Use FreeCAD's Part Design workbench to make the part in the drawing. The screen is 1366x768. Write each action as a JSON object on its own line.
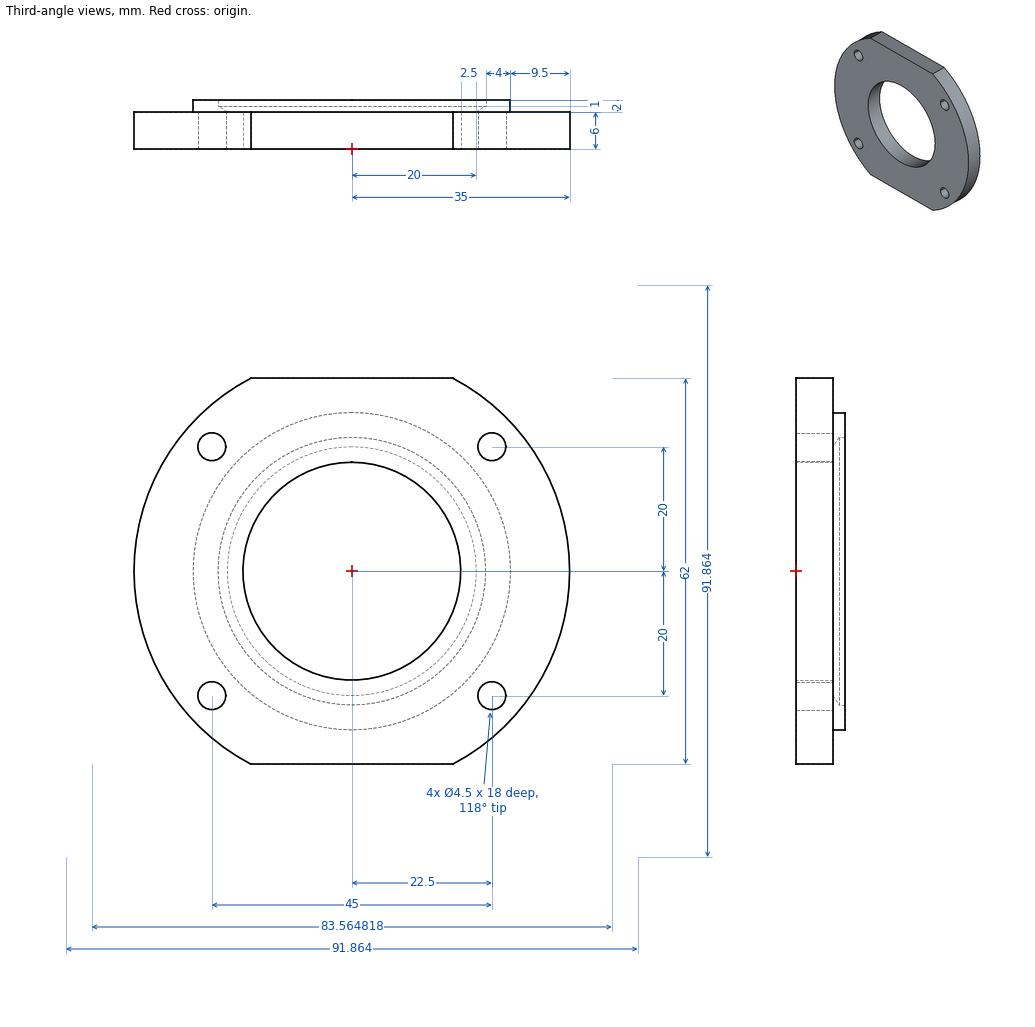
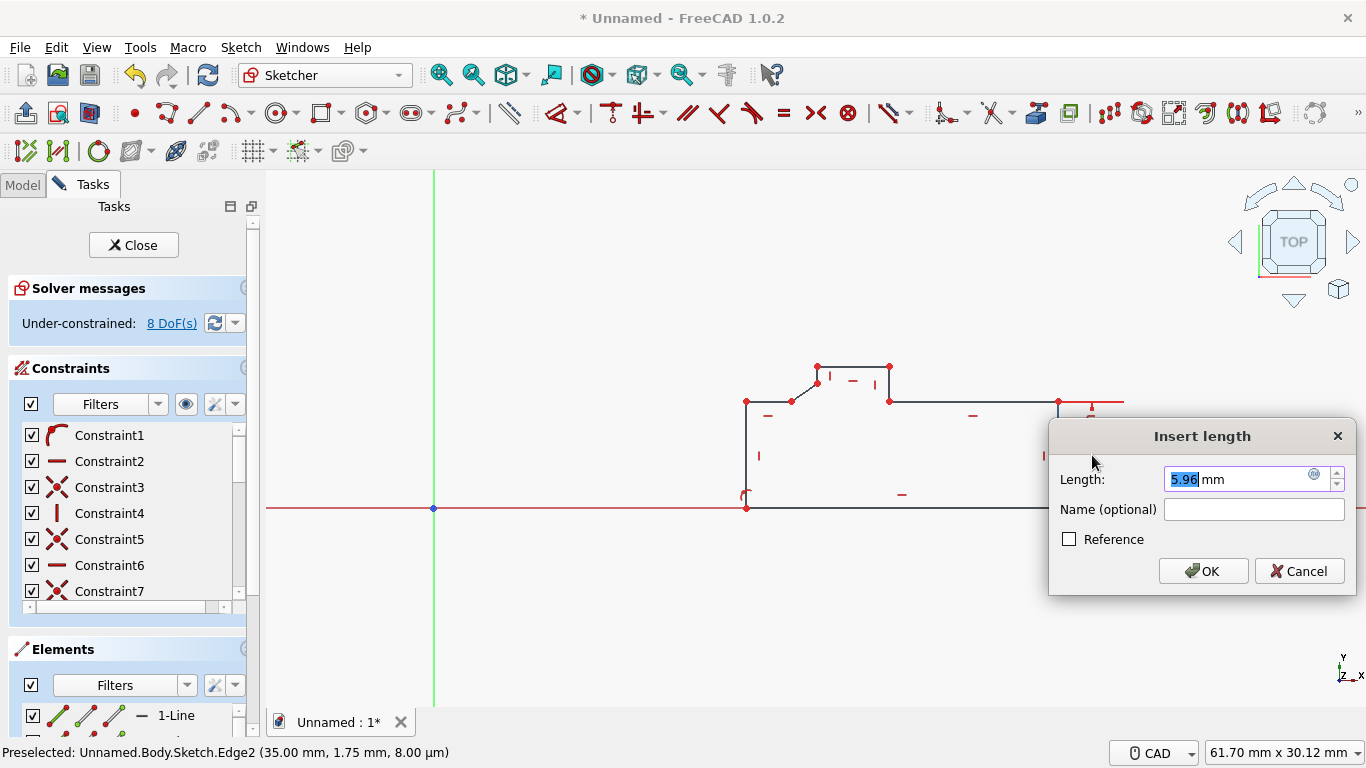
{"action": "type", "text": "6"}
{"action": "key", "text": "Return"}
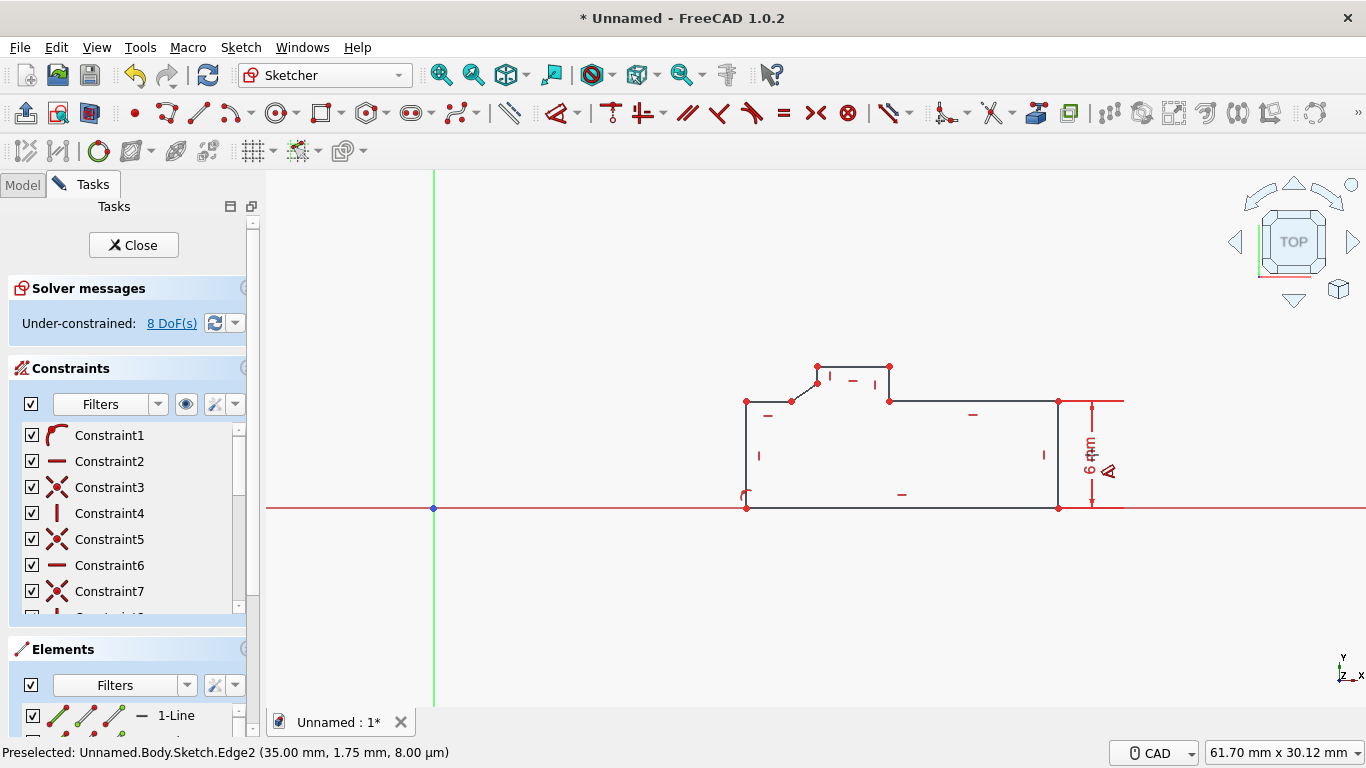
{"action": "scroll", "coordinate": [889, 391], "scroll_direction": "up", "scroll_amount": 2}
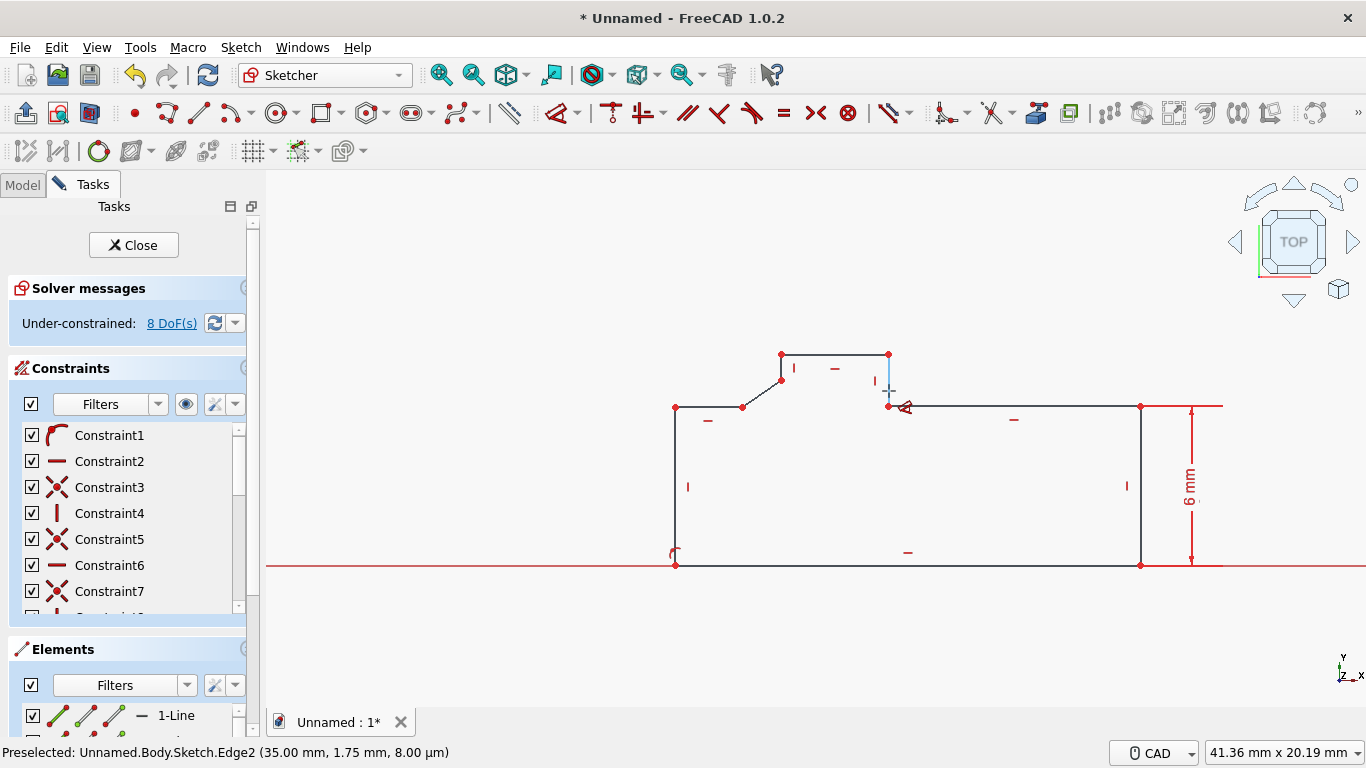
{"action": "left_click", "coordinate": [889, 391]}
{"action": "left_click", "coordinate": [923, 381]}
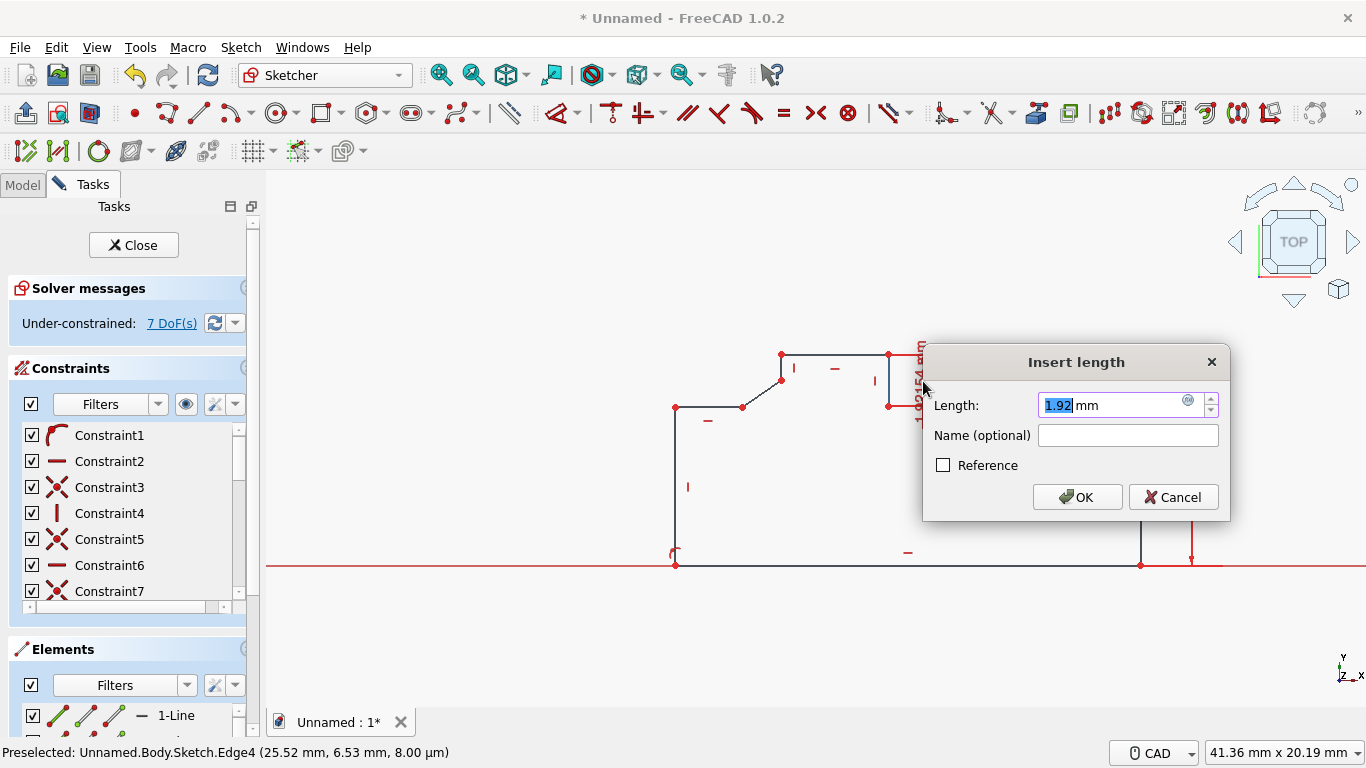
{"action": "type", "text": "2"}
{"action": "key", "text": "Return"}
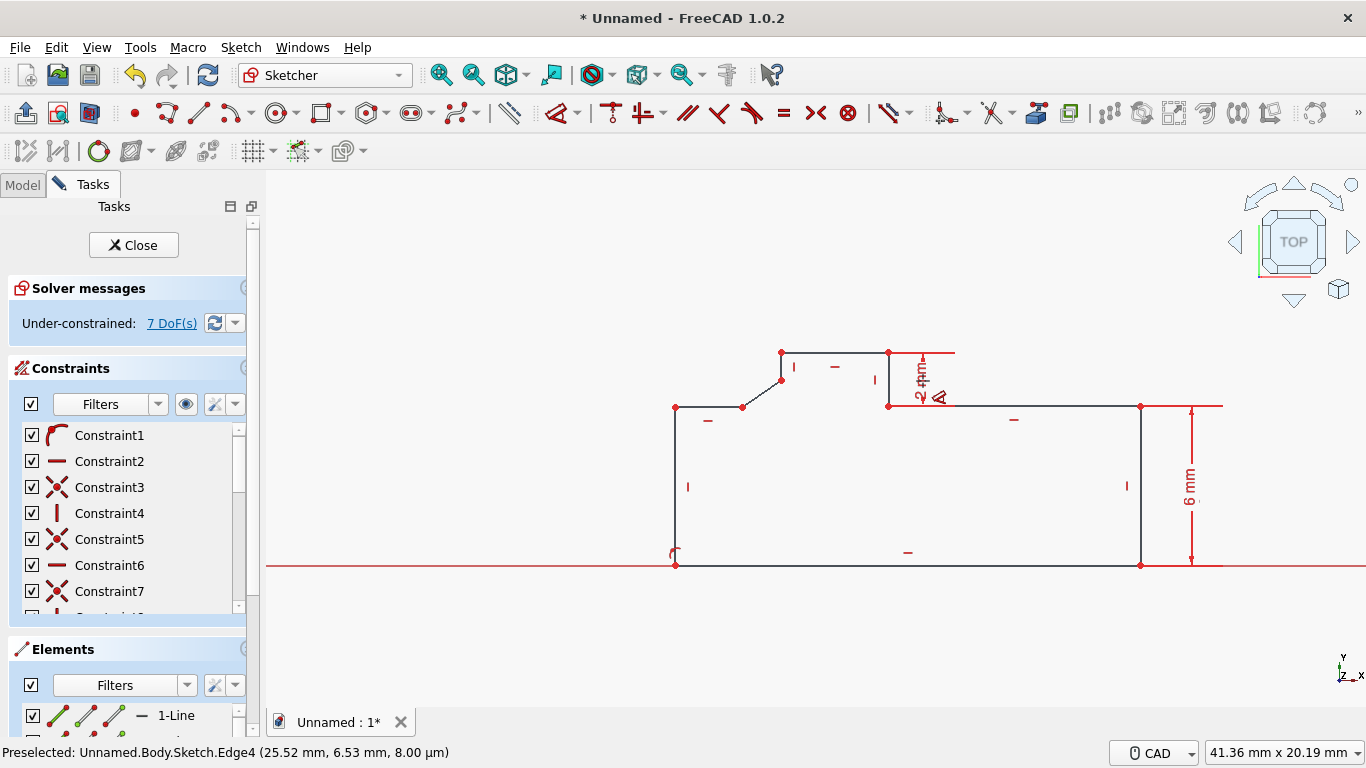
{"action": "left_click", "coordinate": [856, 353]}
{"action": "left_click", "coordinate": [835, 319]}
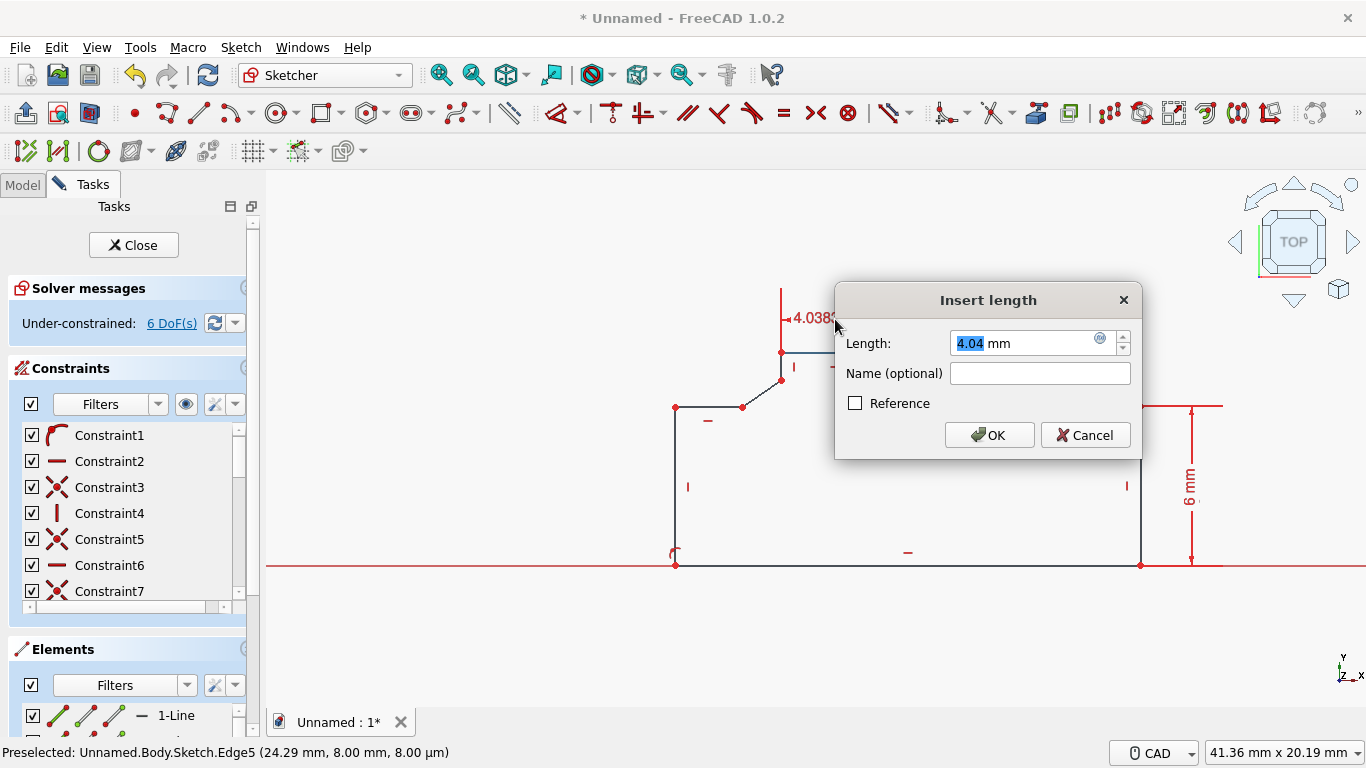
{"action": "type", "text": "4"}
{"action": "key", "text": "Return"}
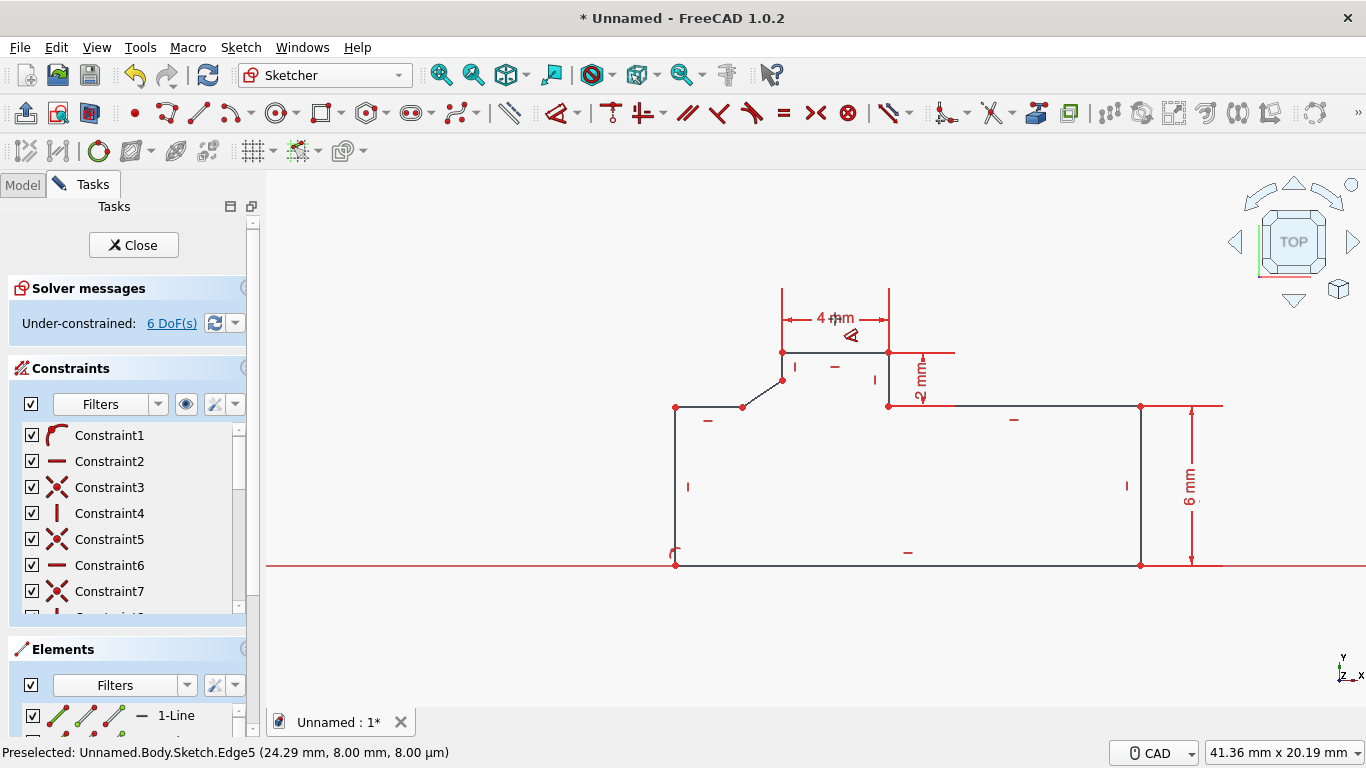
{"action": "scroll", "coordinate": [782, 364], "scroll_direction": "up", "scroll_amount": 3}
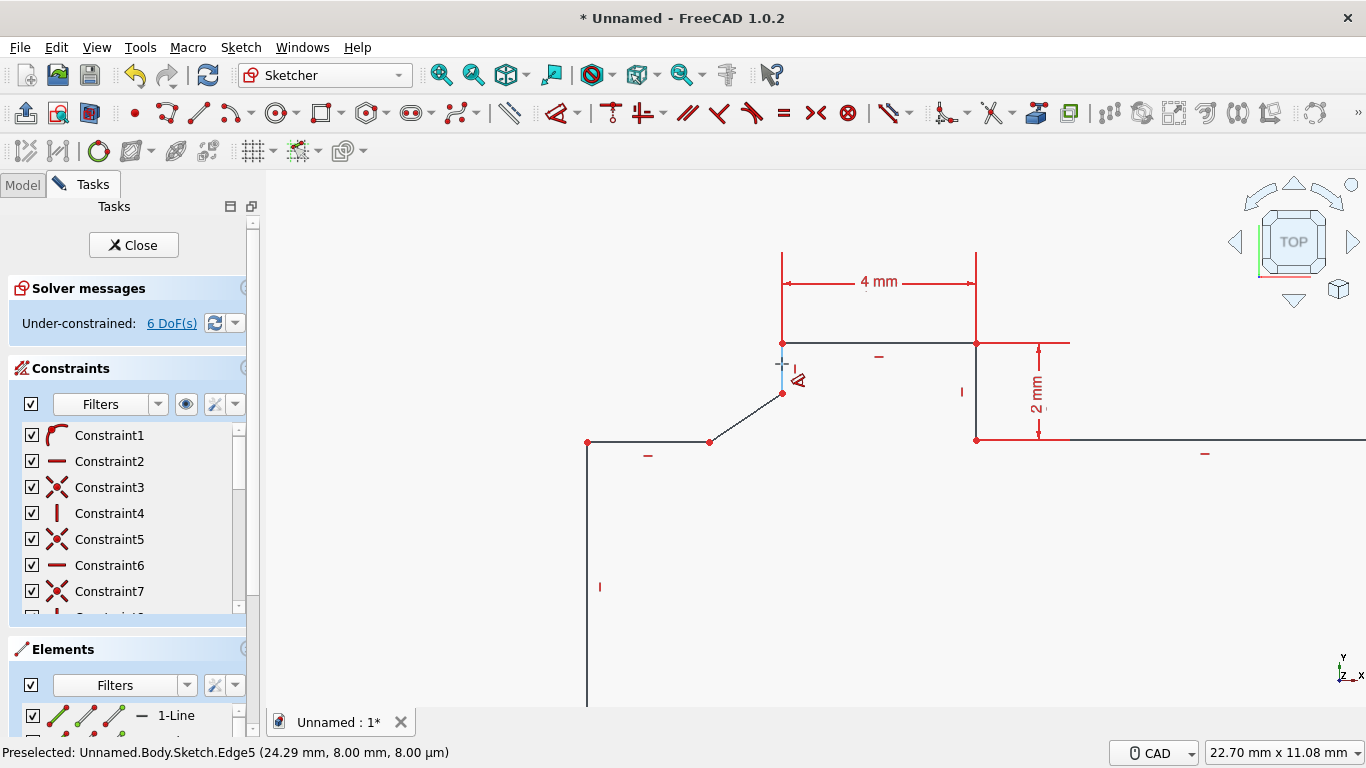
{"action": "left_click", "coordinate": [782, 363]}
{"action": "left_click", "coordinate": [816, 368]}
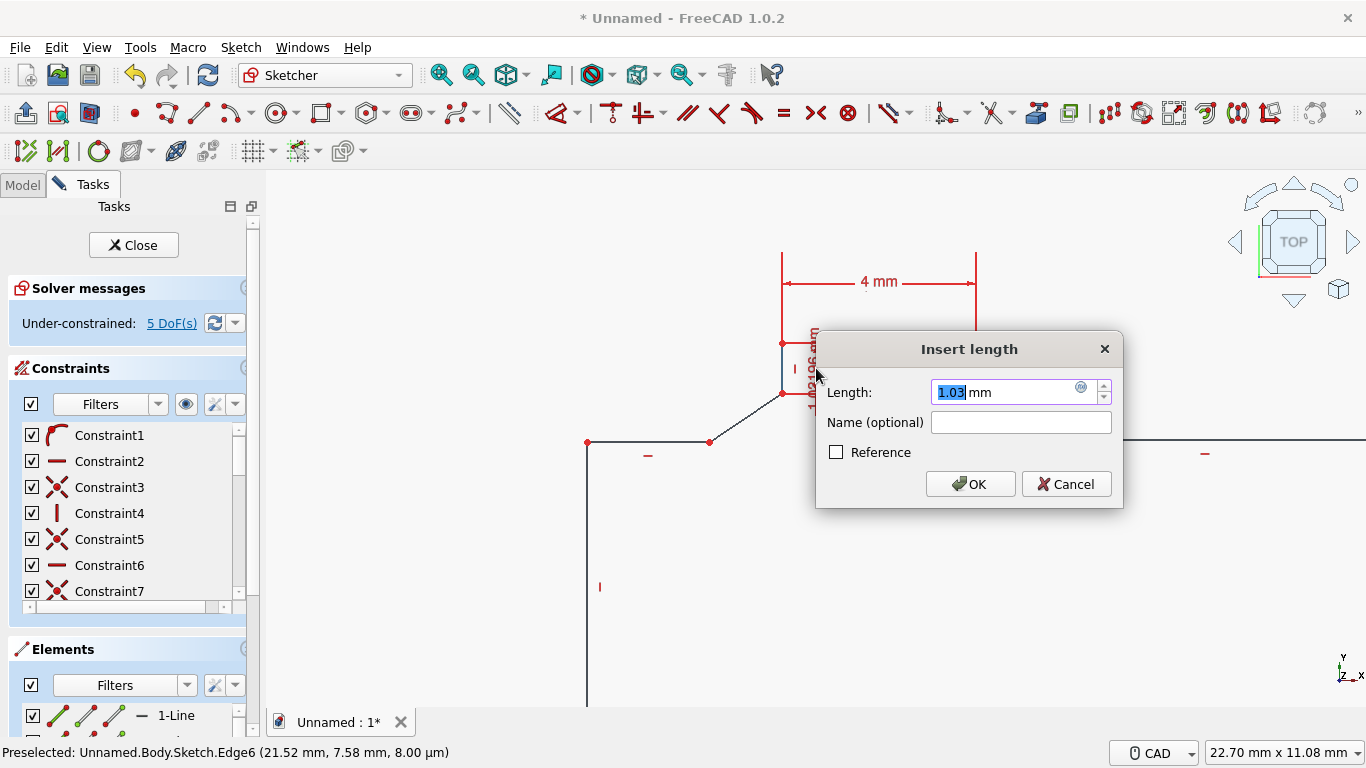
{"action": "type", "text": "1"}
{"action": "key", "text": "Return"}